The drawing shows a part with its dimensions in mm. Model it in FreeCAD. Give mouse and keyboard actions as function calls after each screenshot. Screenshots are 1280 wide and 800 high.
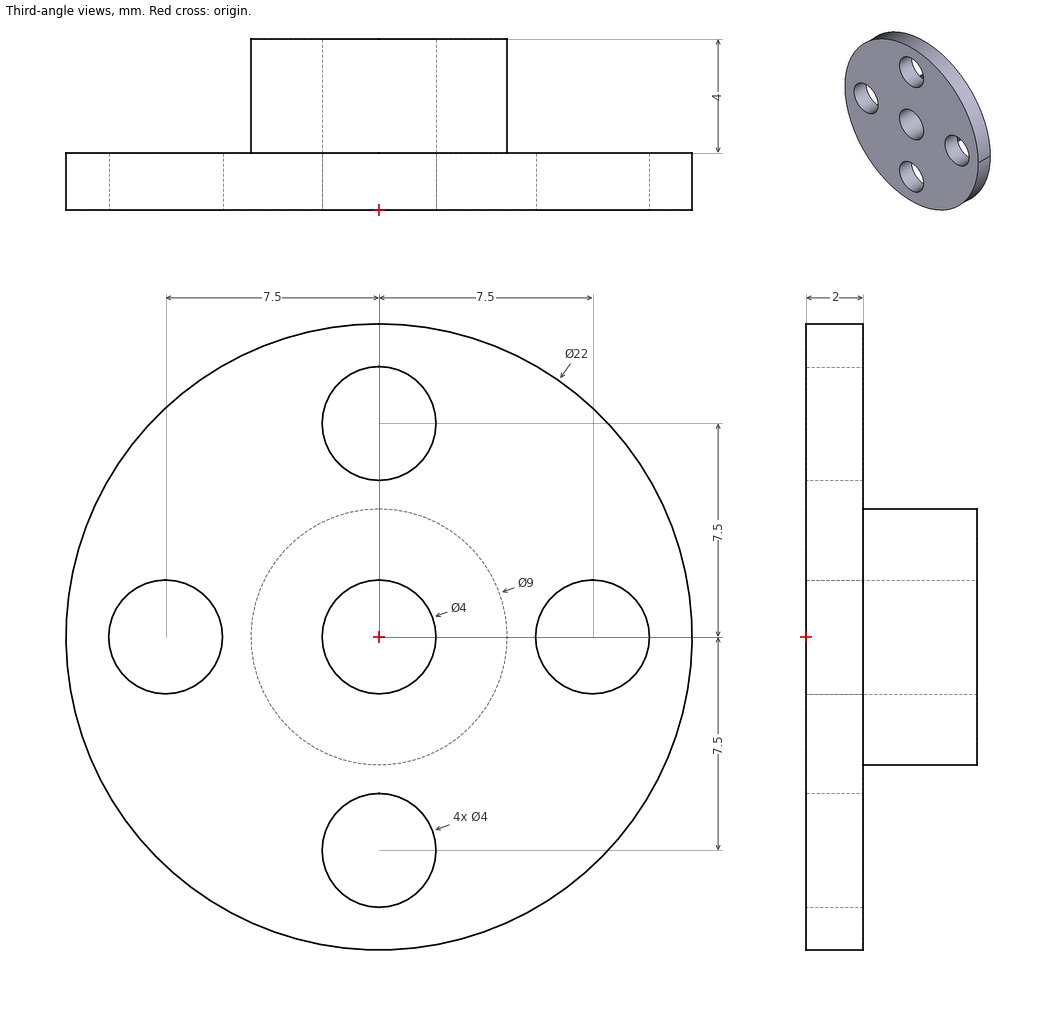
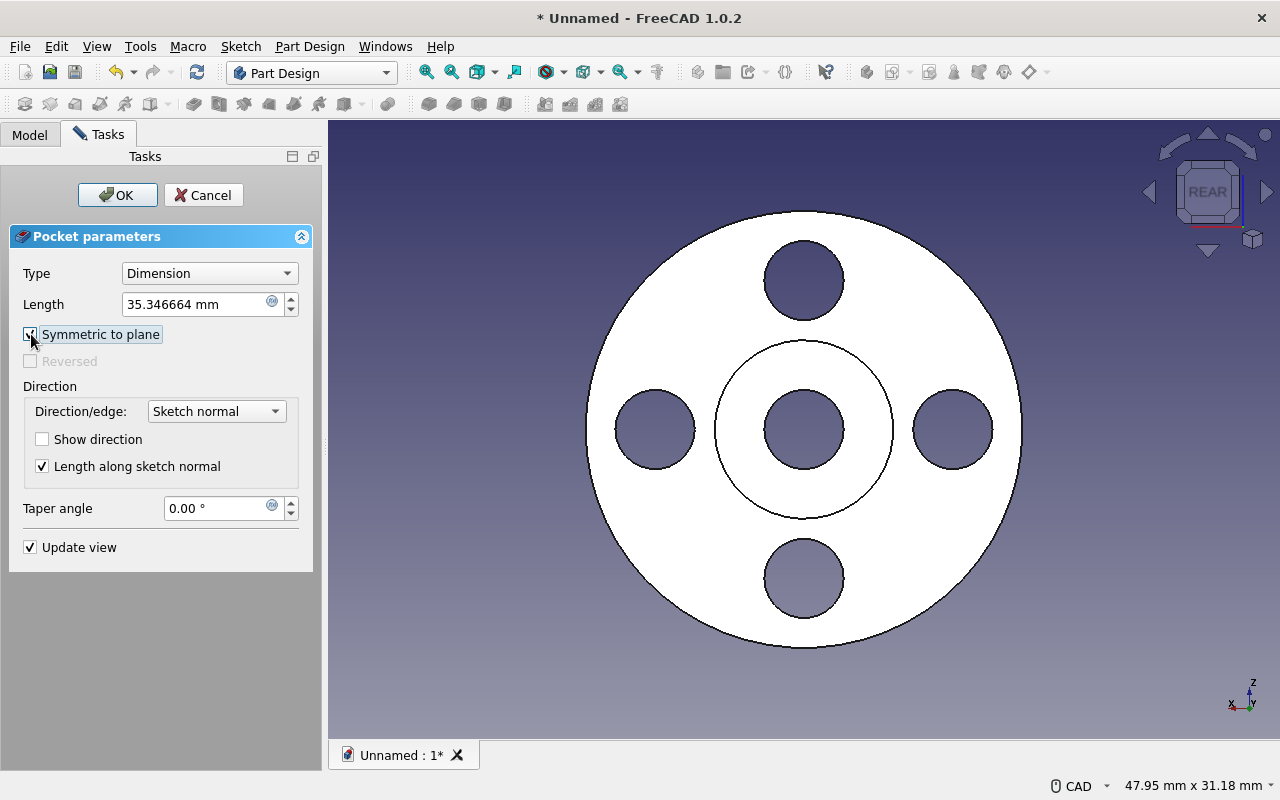
click(118, 195)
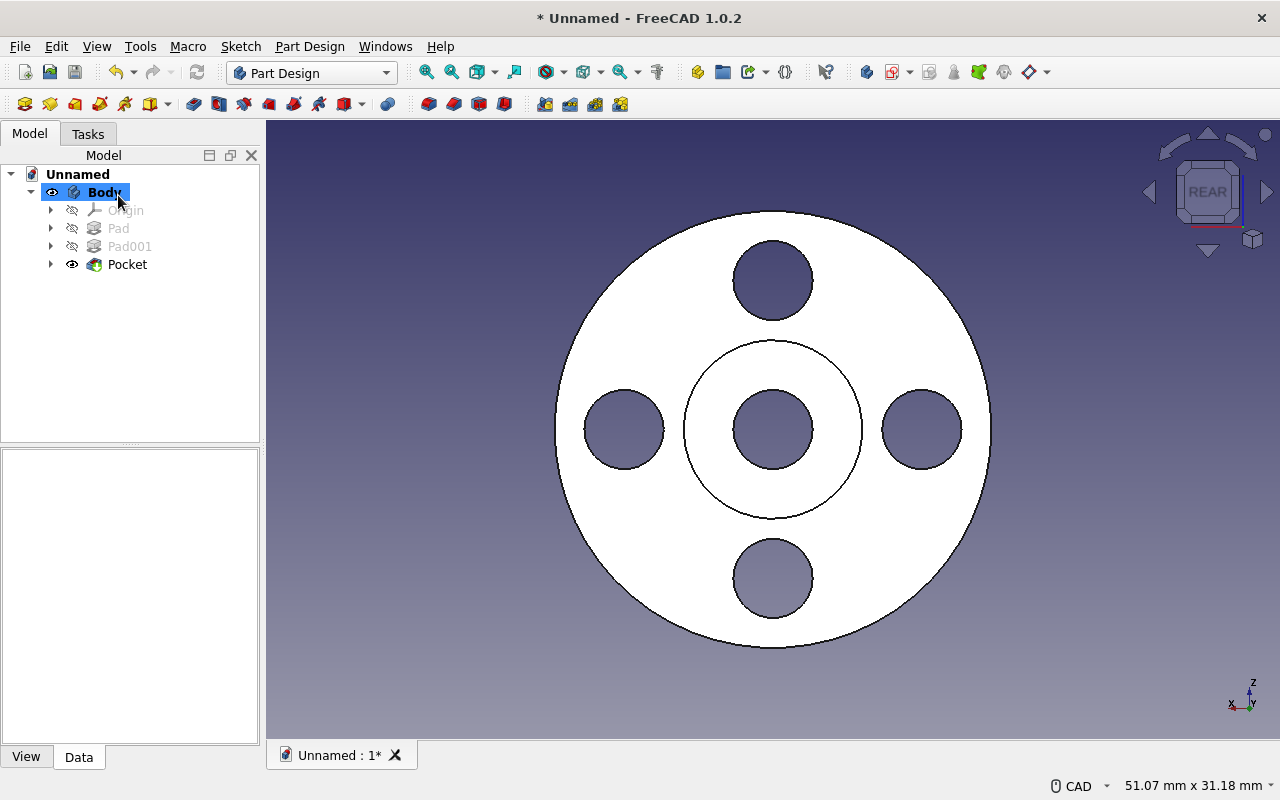
key(0)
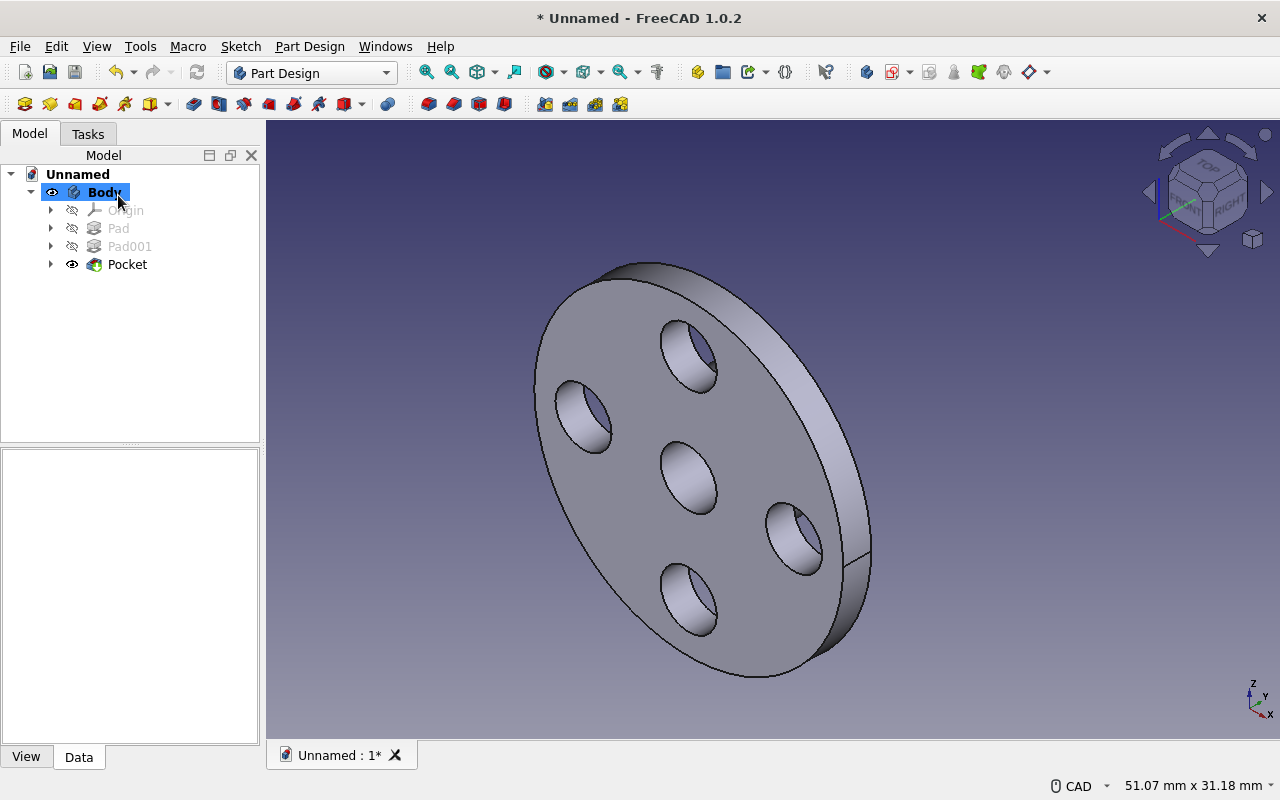
click(427, 72)